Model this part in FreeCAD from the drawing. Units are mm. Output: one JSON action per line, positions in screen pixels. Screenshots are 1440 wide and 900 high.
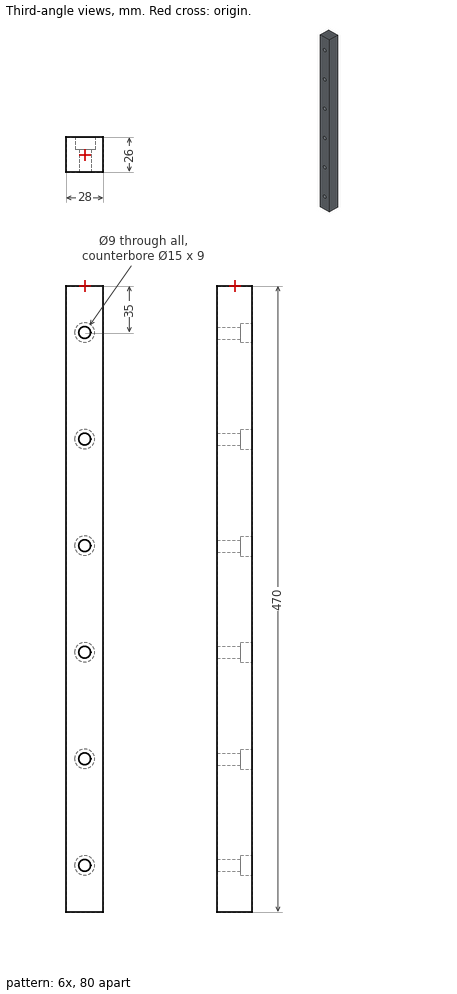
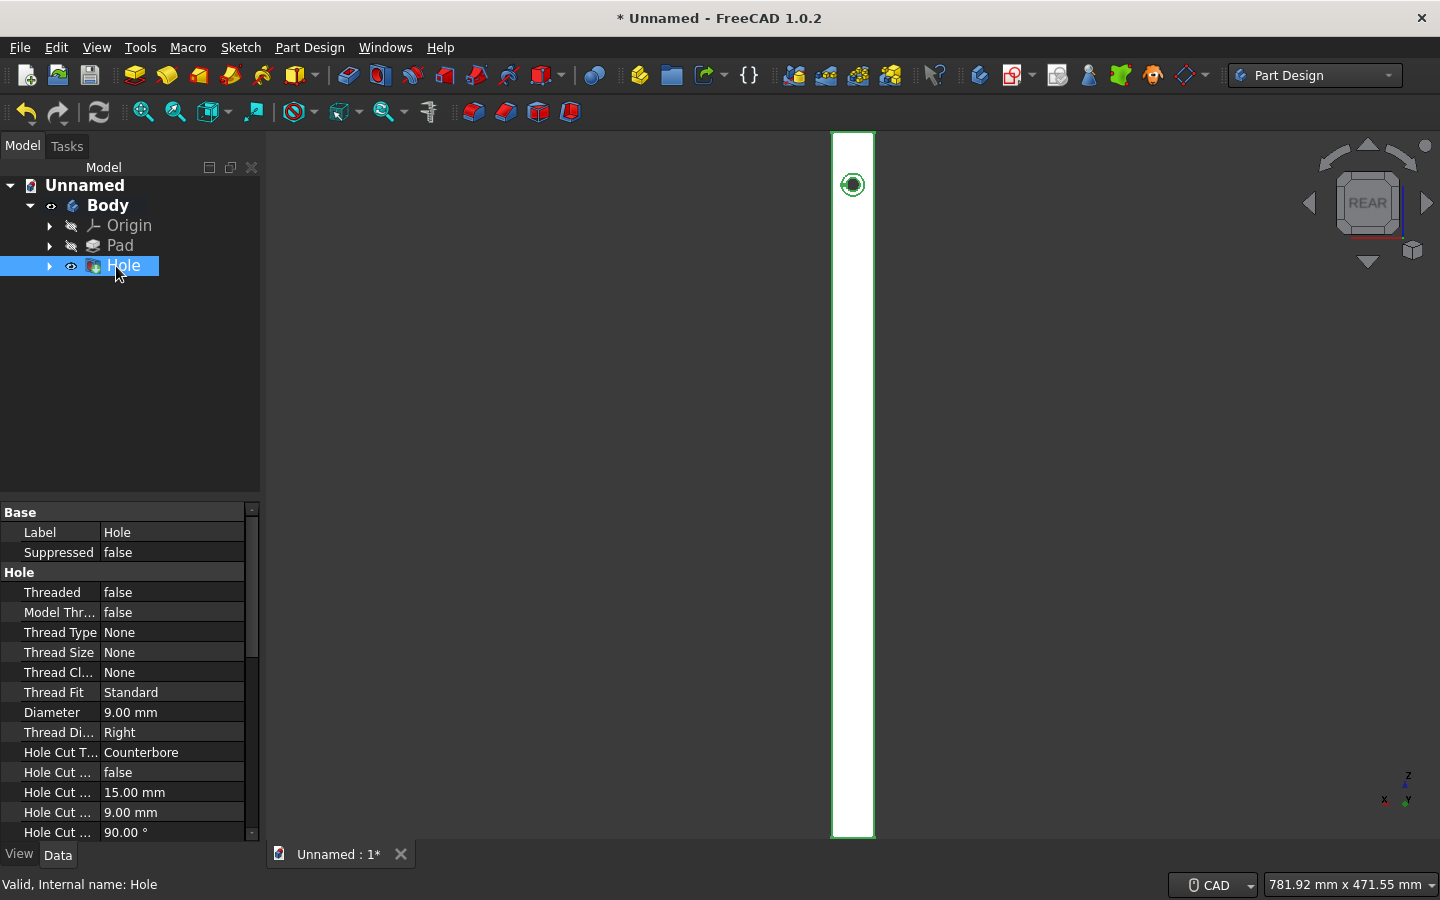
{"action": "left_click", "coordinate": [826, 76]}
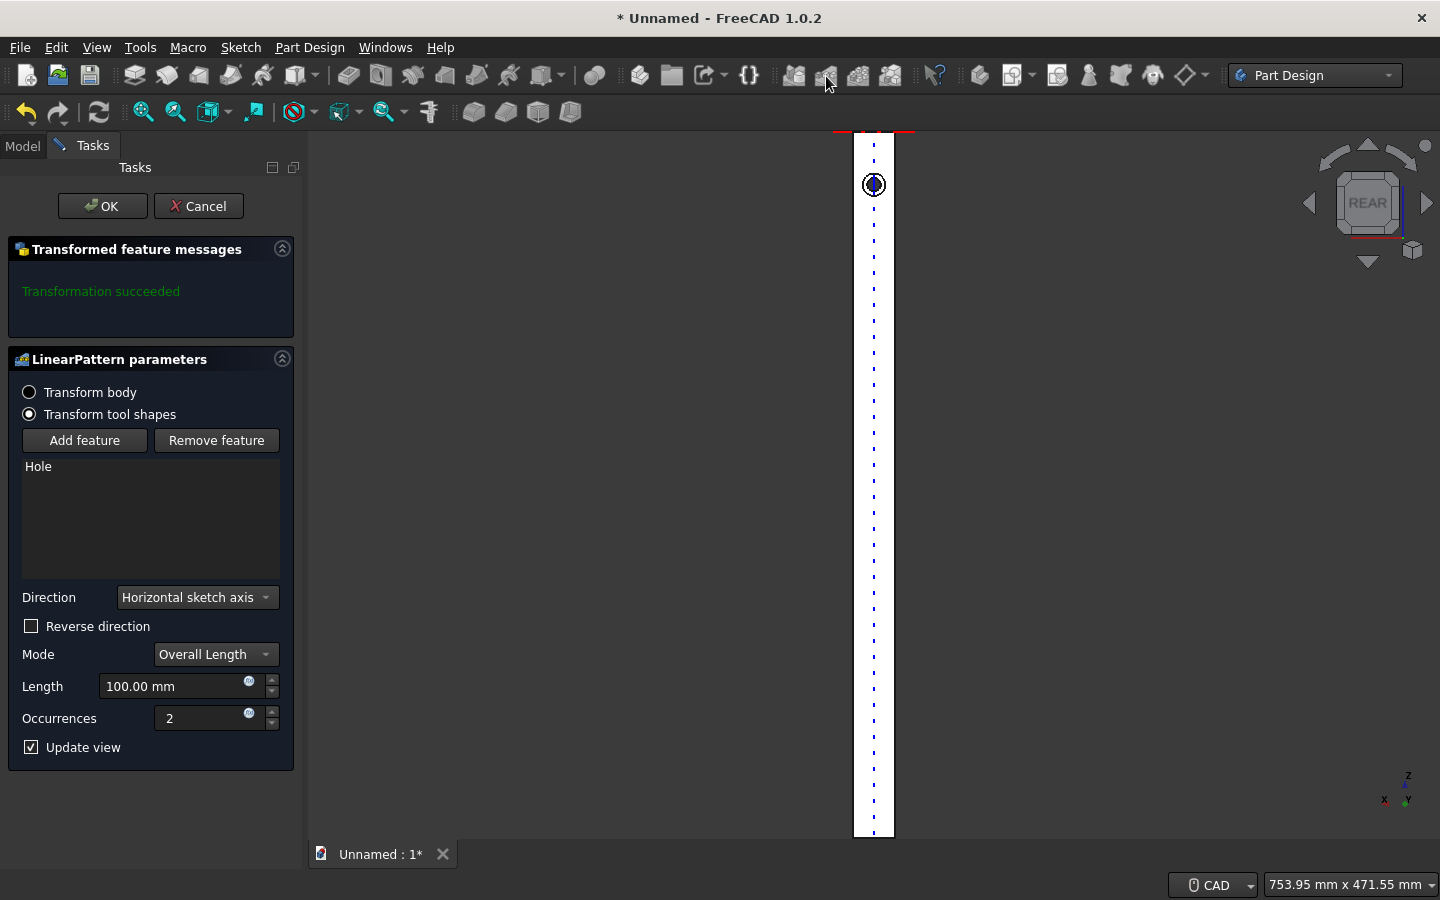
{"action": "left_click", "coordinate": [198, 598]}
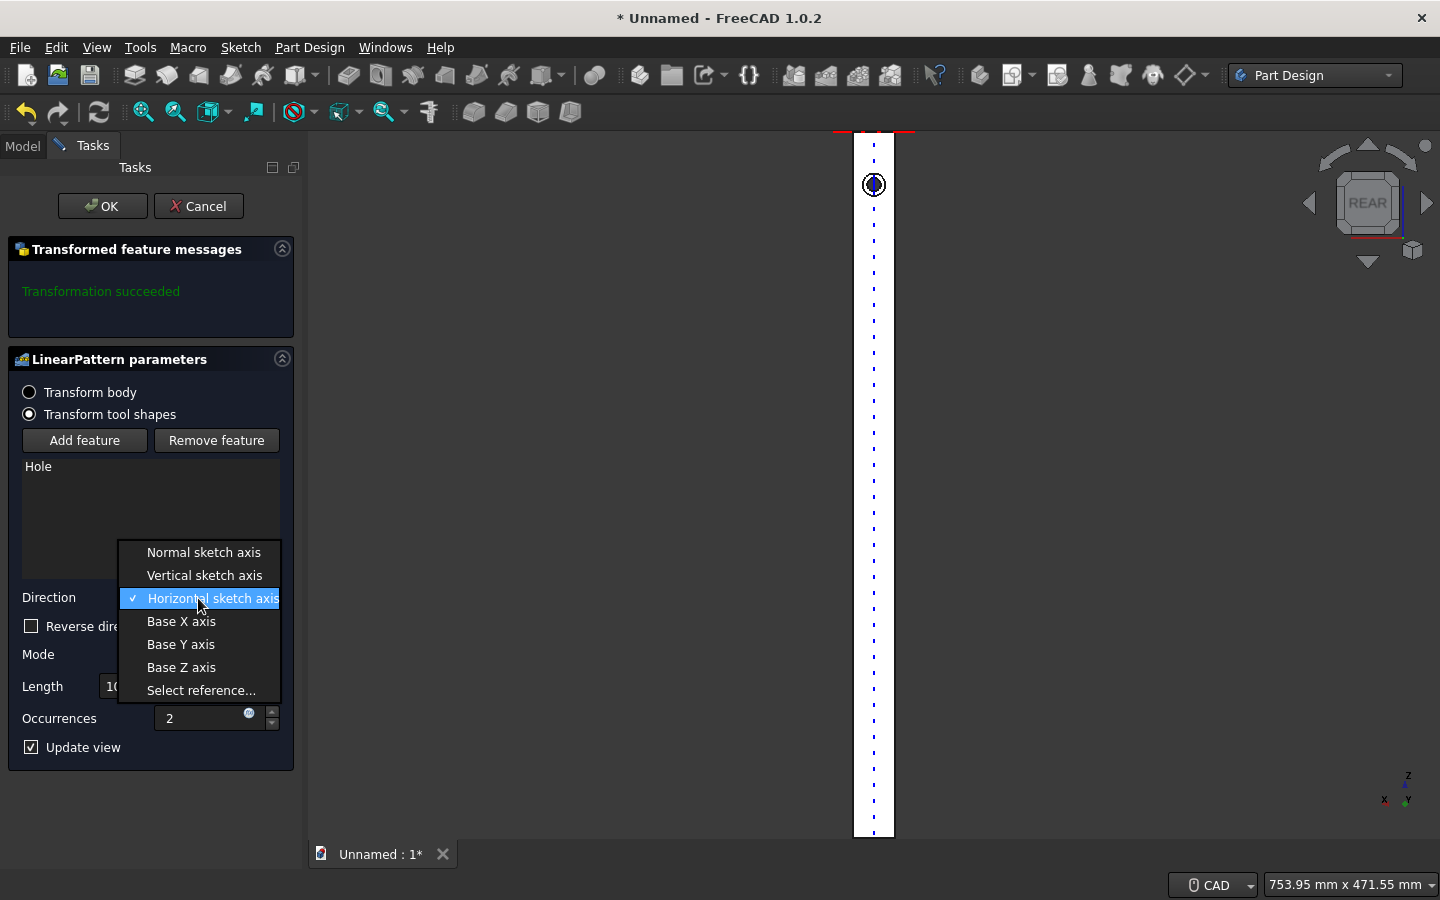
{"action": "left_click", "coordinate": [198, 668]}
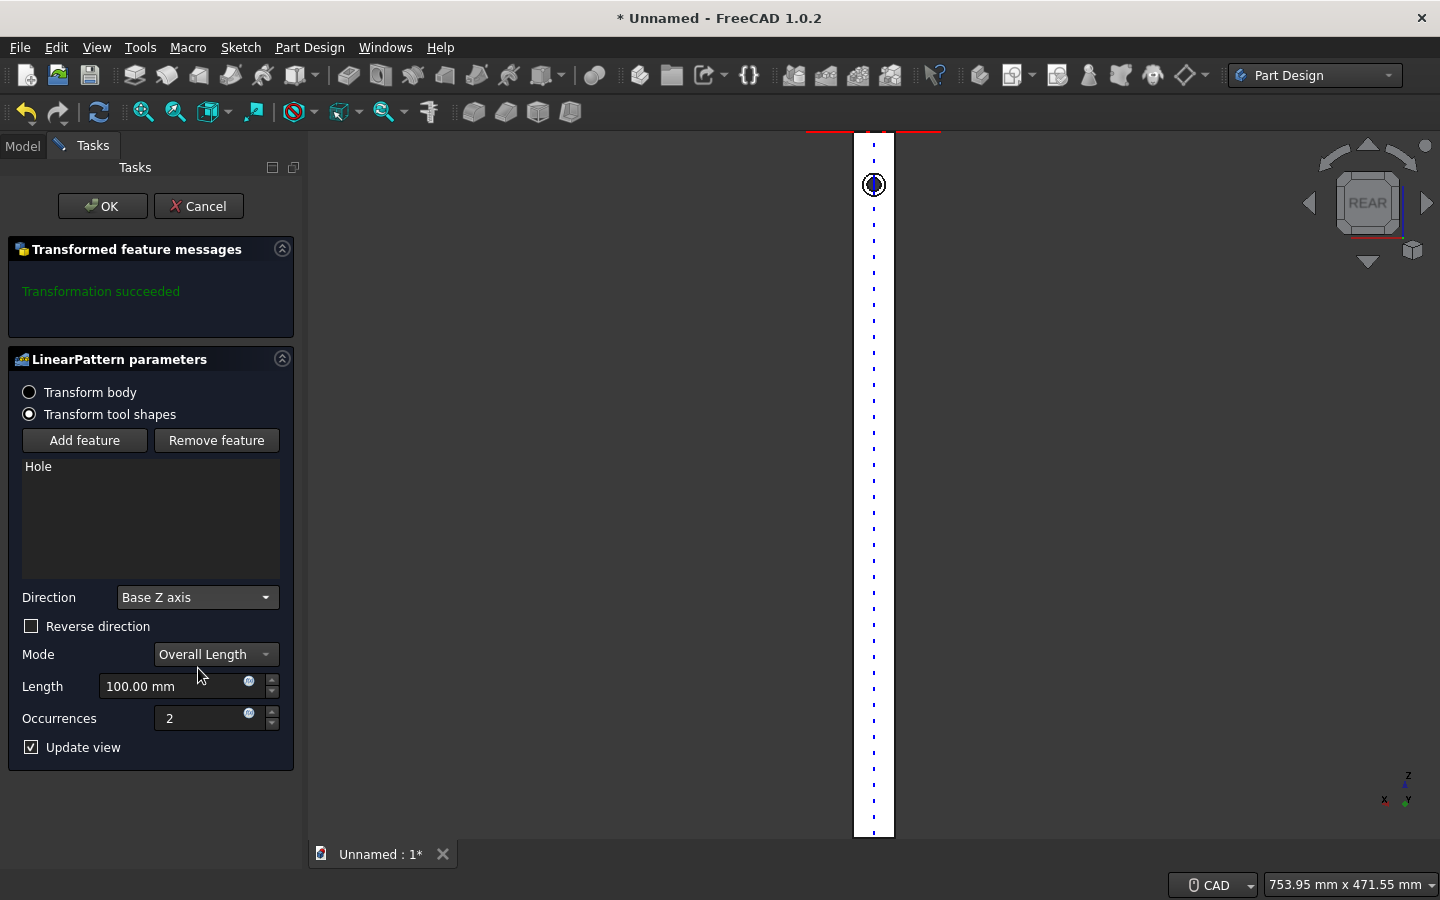
{"action": "left_click", "coordinate": [217, 654]}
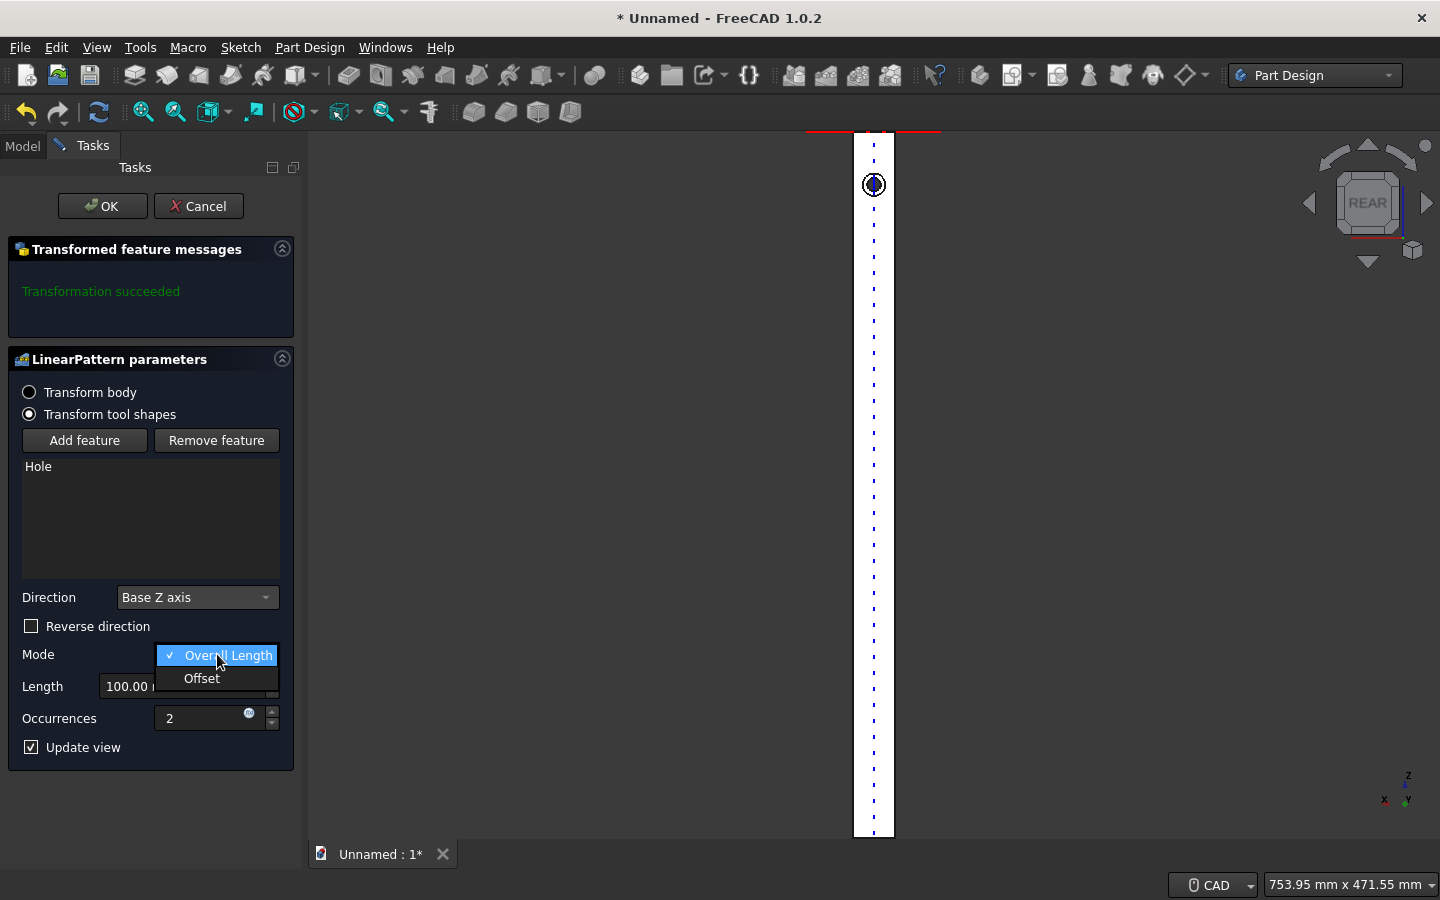
{"action": "left_click", "coordinate": [216, 678]}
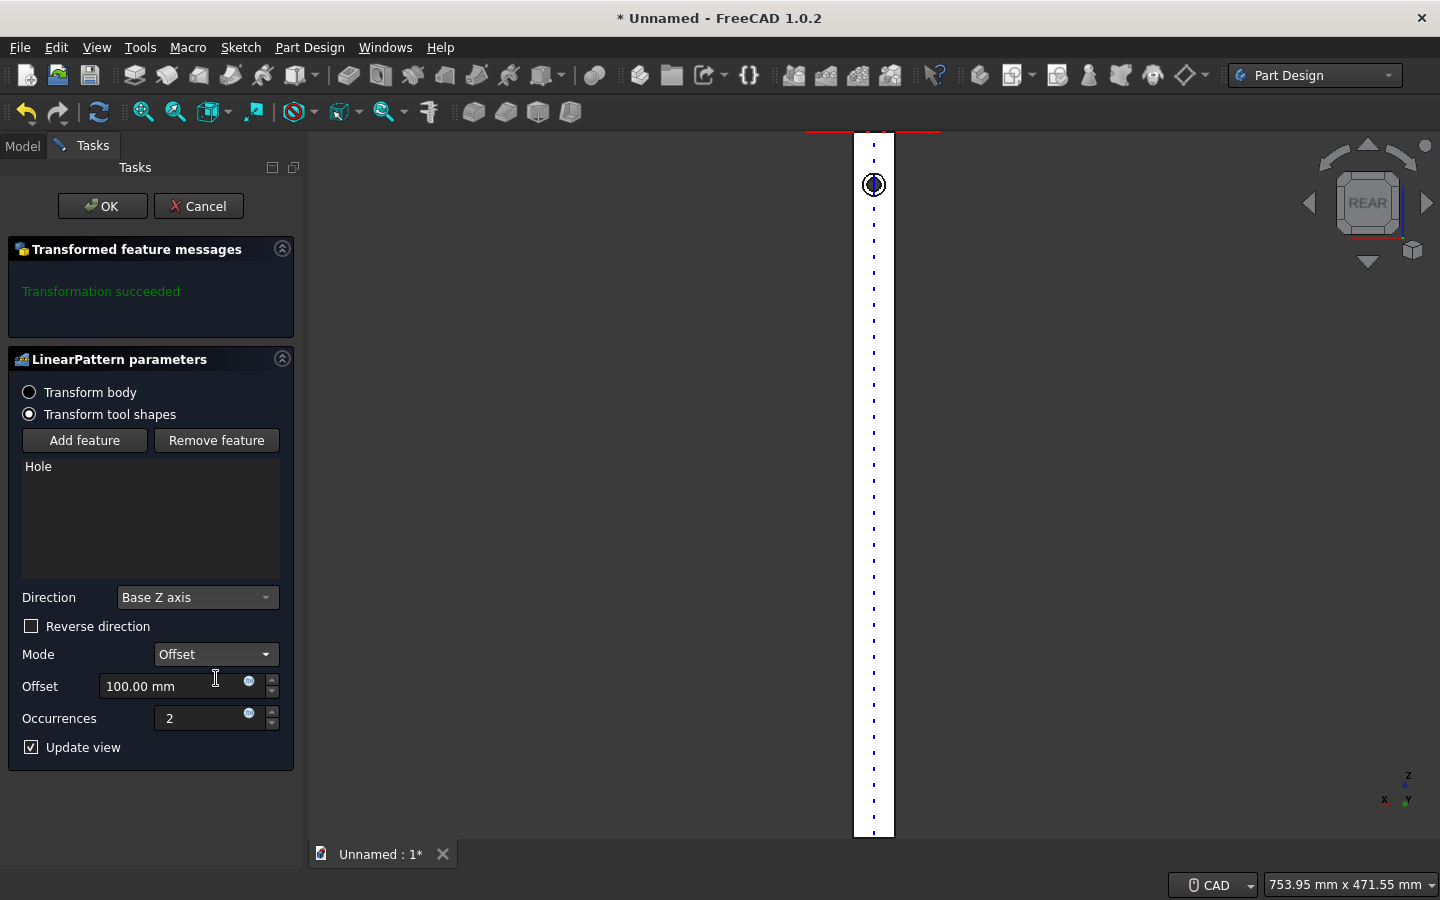
{"action": "triple_click", "coordinate": [182, 686]}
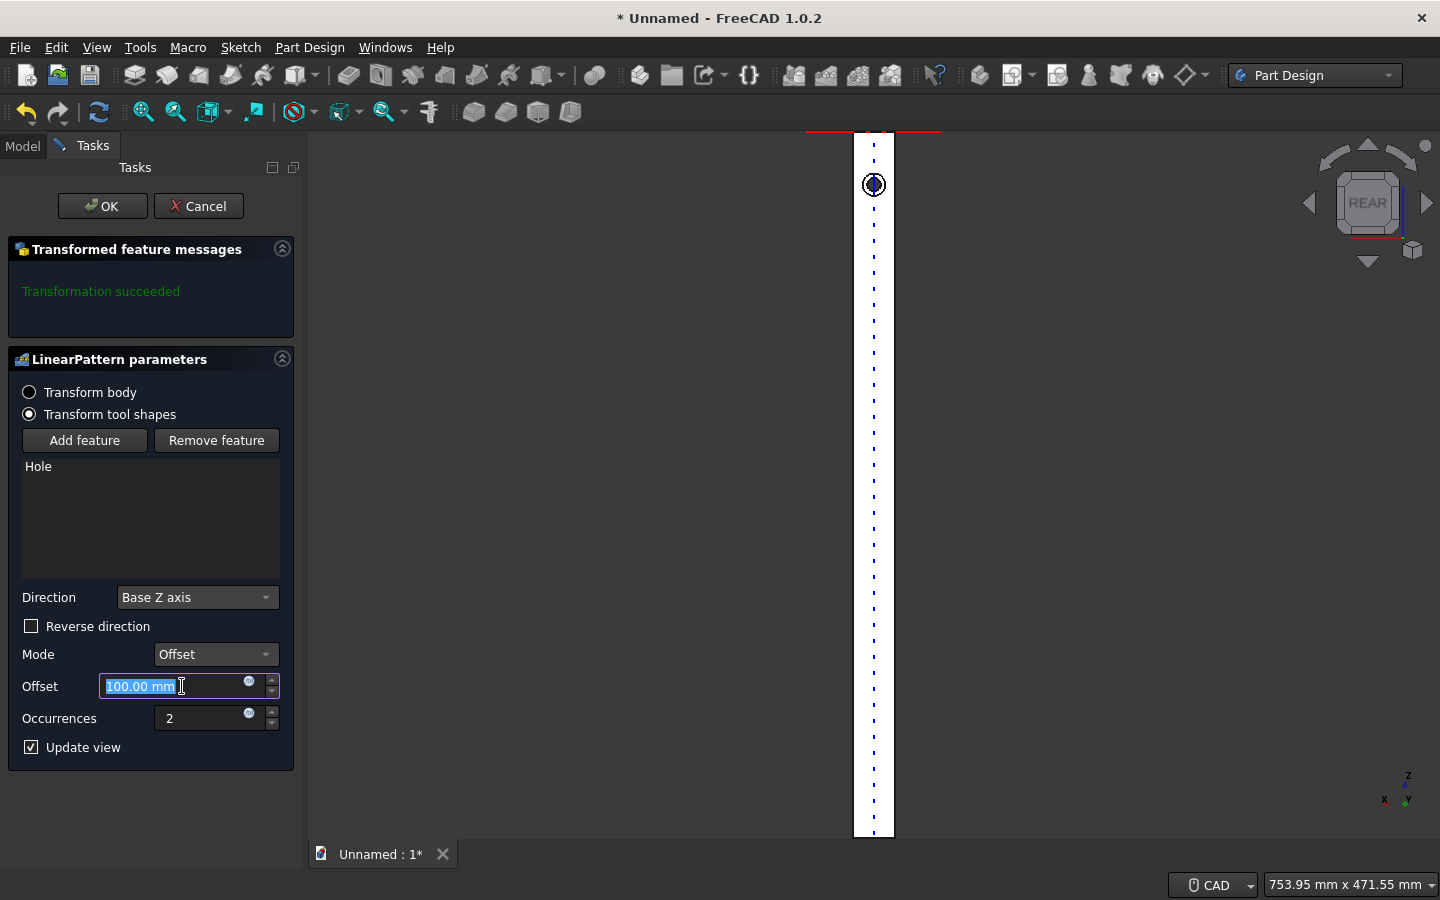
{"action": "type", "text": "80"}
{"action": "key", "text": "Tab"}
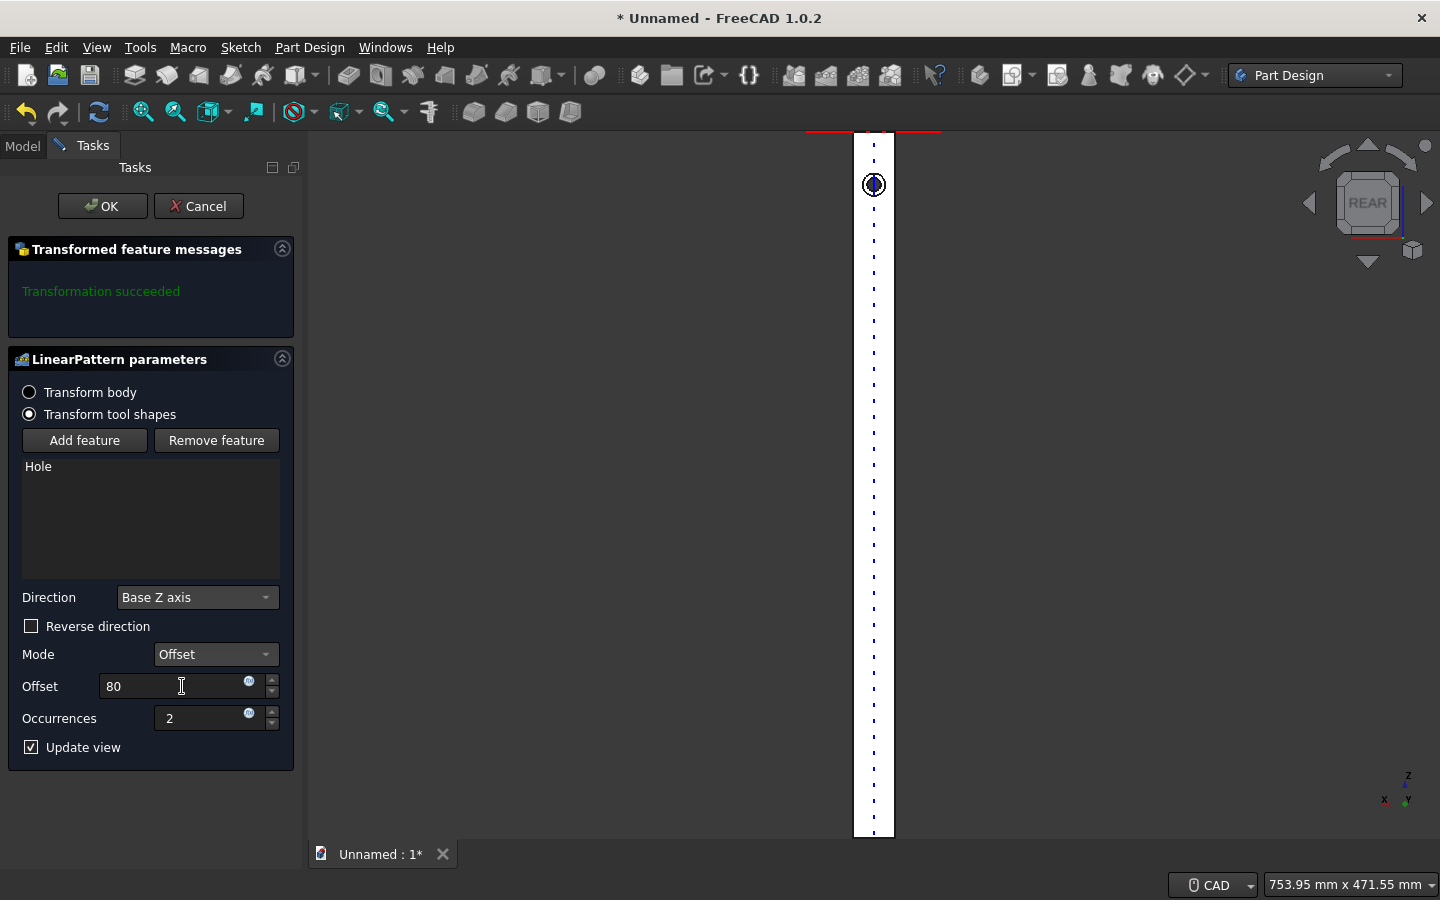
{"action": "triple_click", "coordinate": [209, 718]}